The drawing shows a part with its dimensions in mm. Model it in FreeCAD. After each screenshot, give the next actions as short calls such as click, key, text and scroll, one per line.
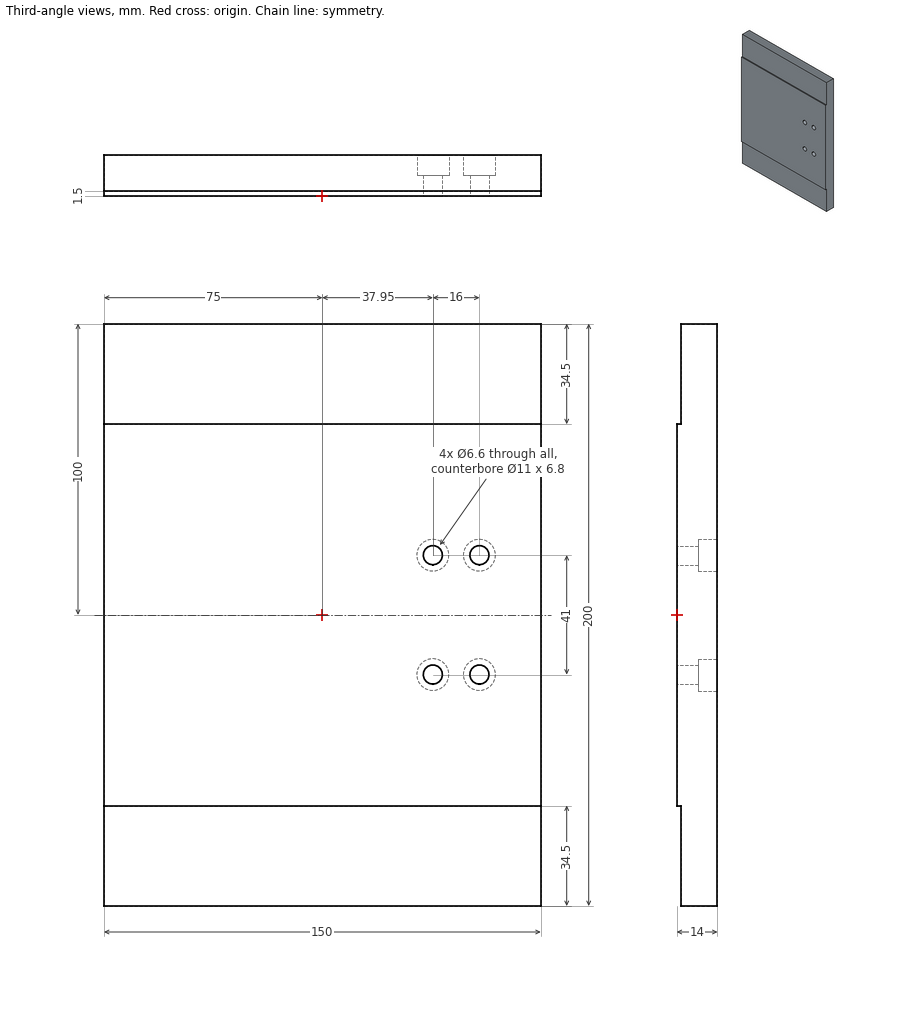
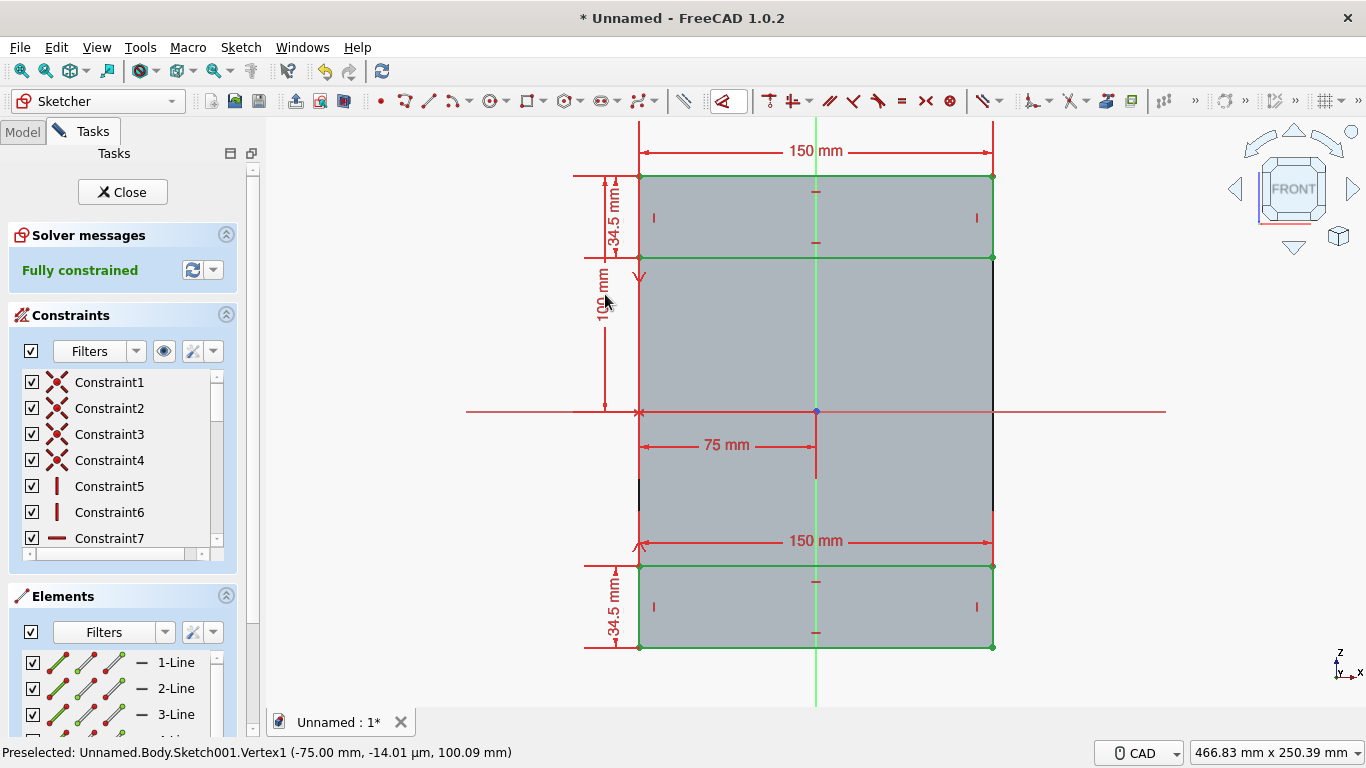
click(123, 192)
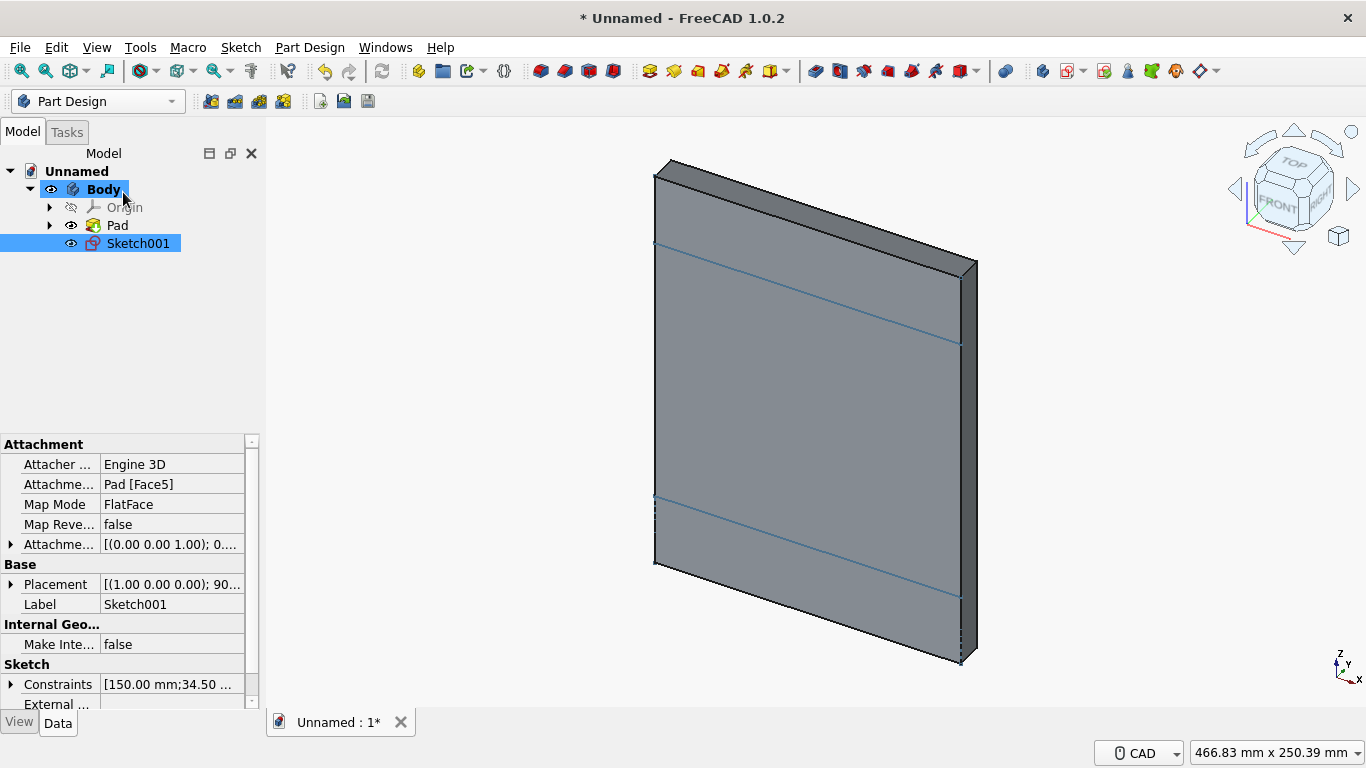
click(816, 72)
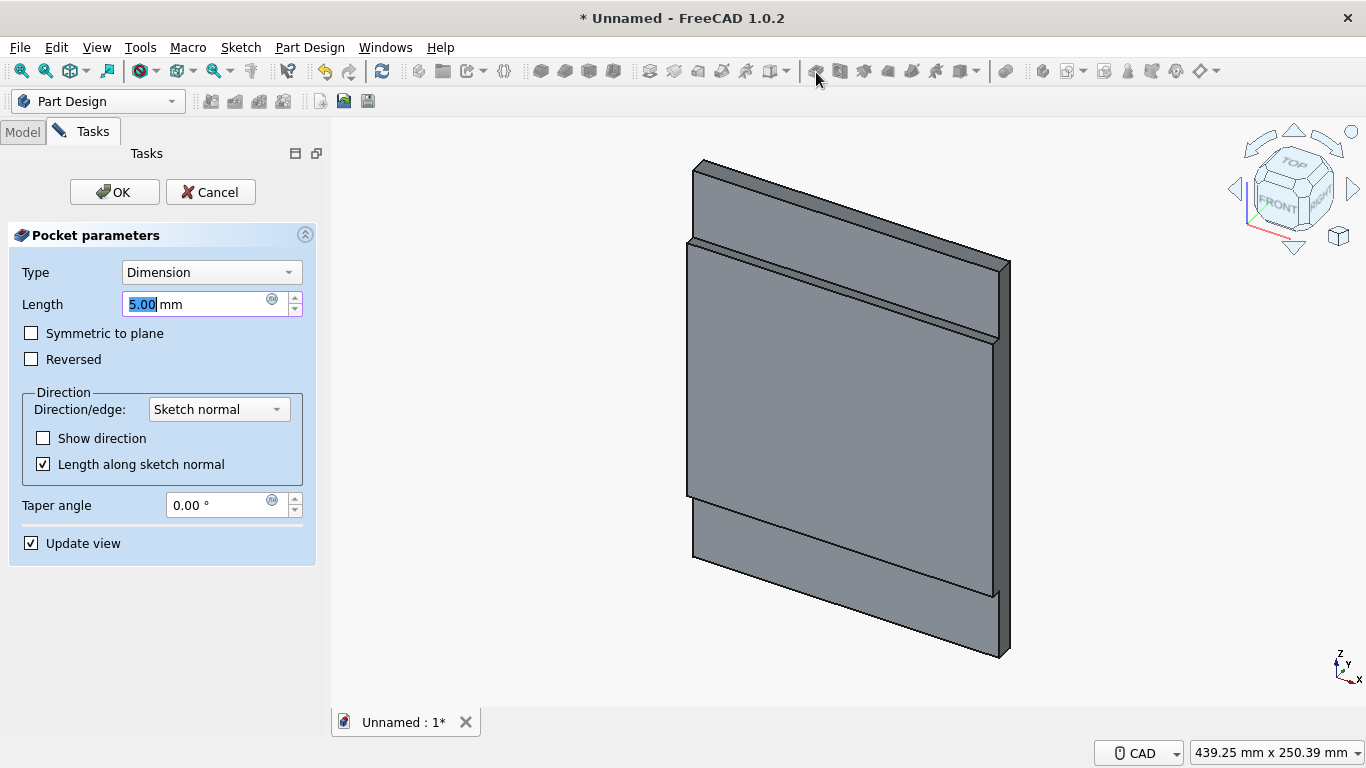
text(1.5)
key(Tab)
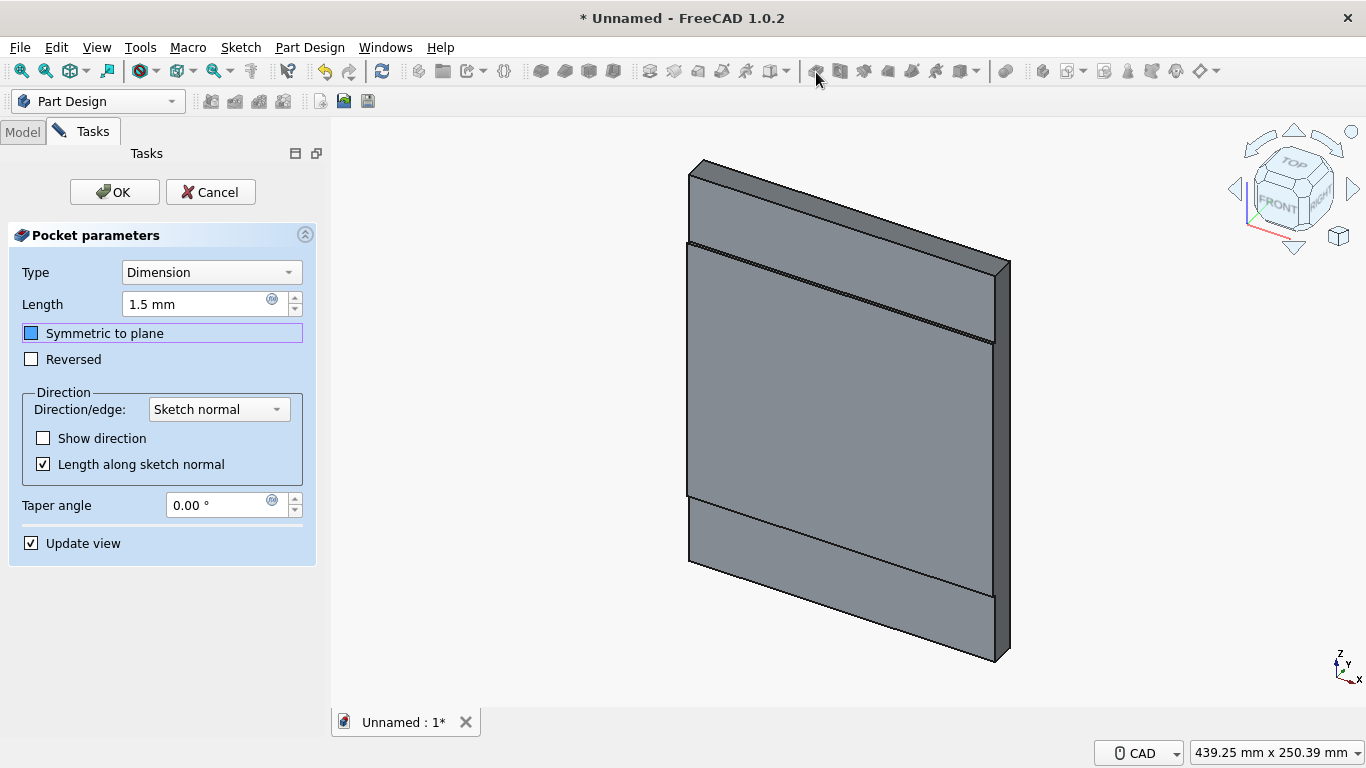
click(115, 192)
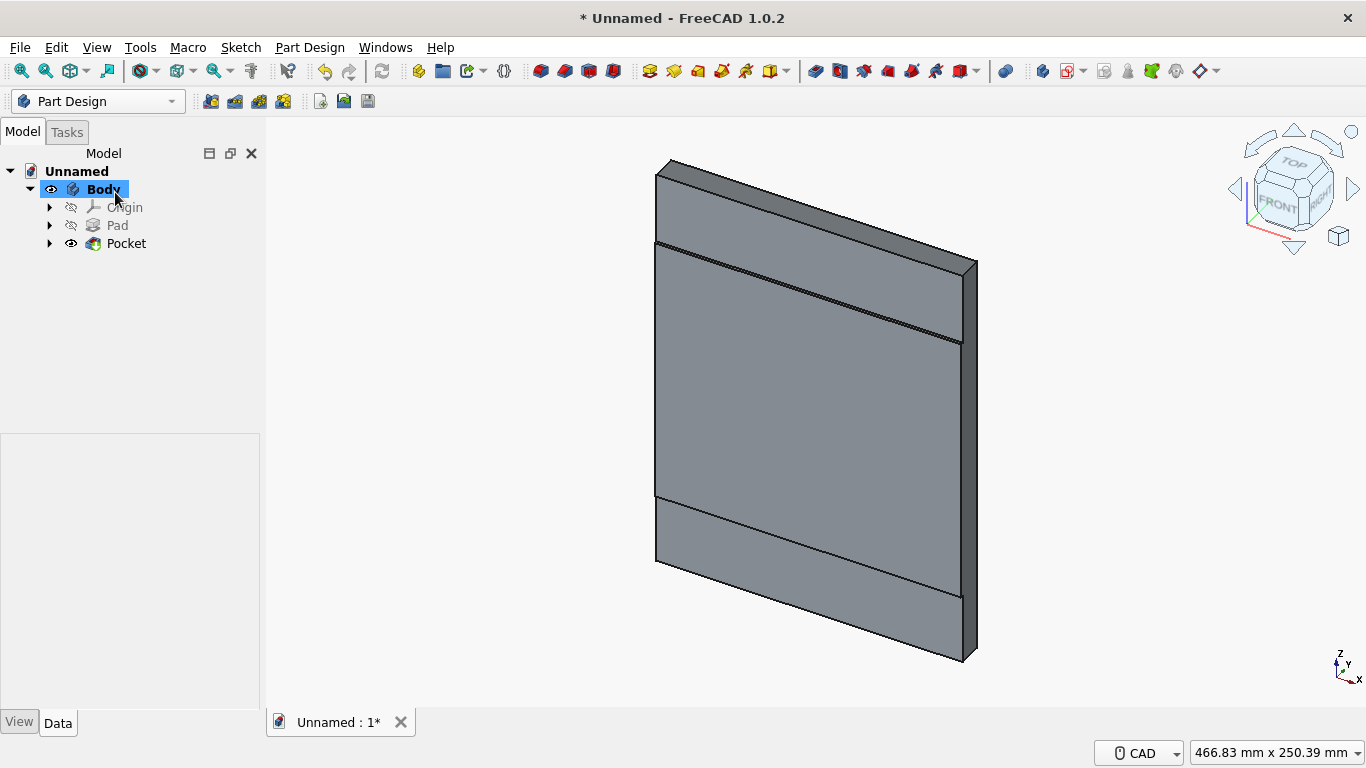
key(4)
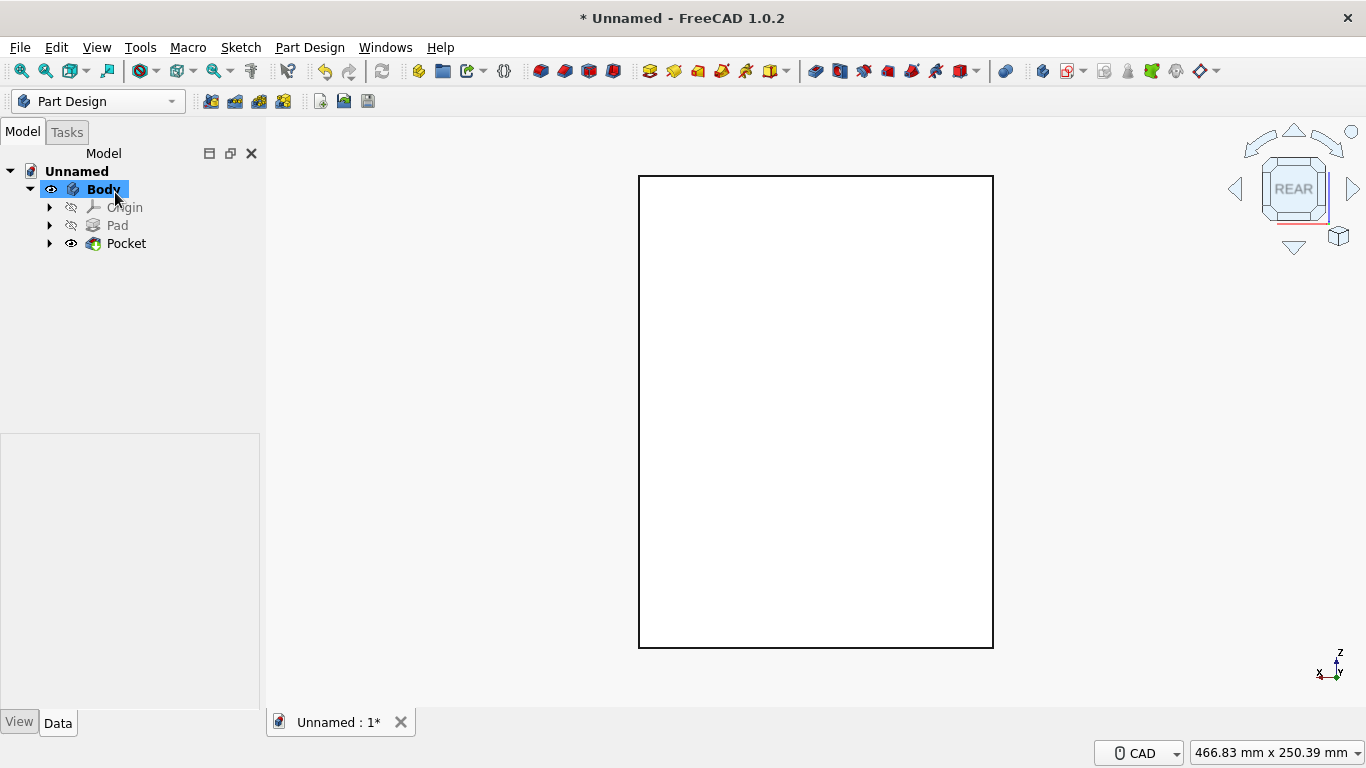
click(816, 411)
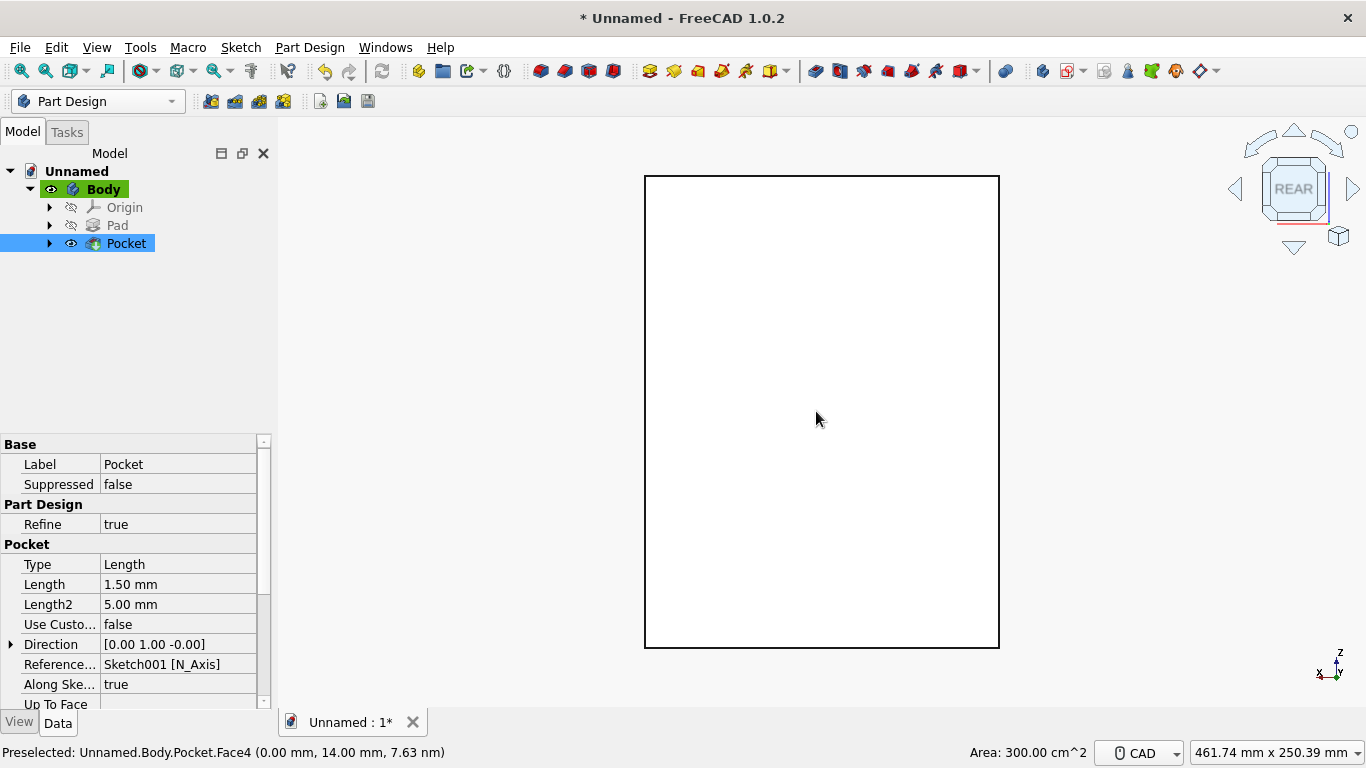
click(1068, 72)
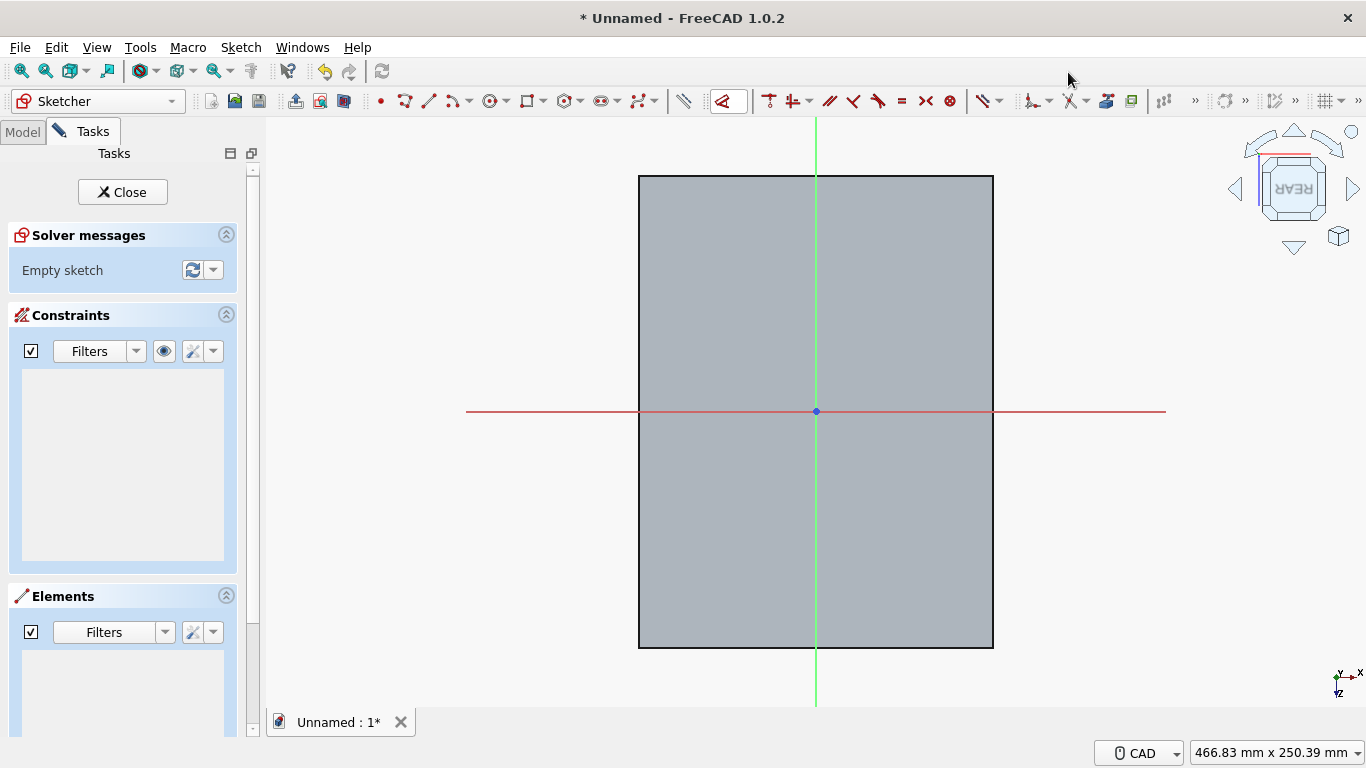
scroll(942, 412, up, 6)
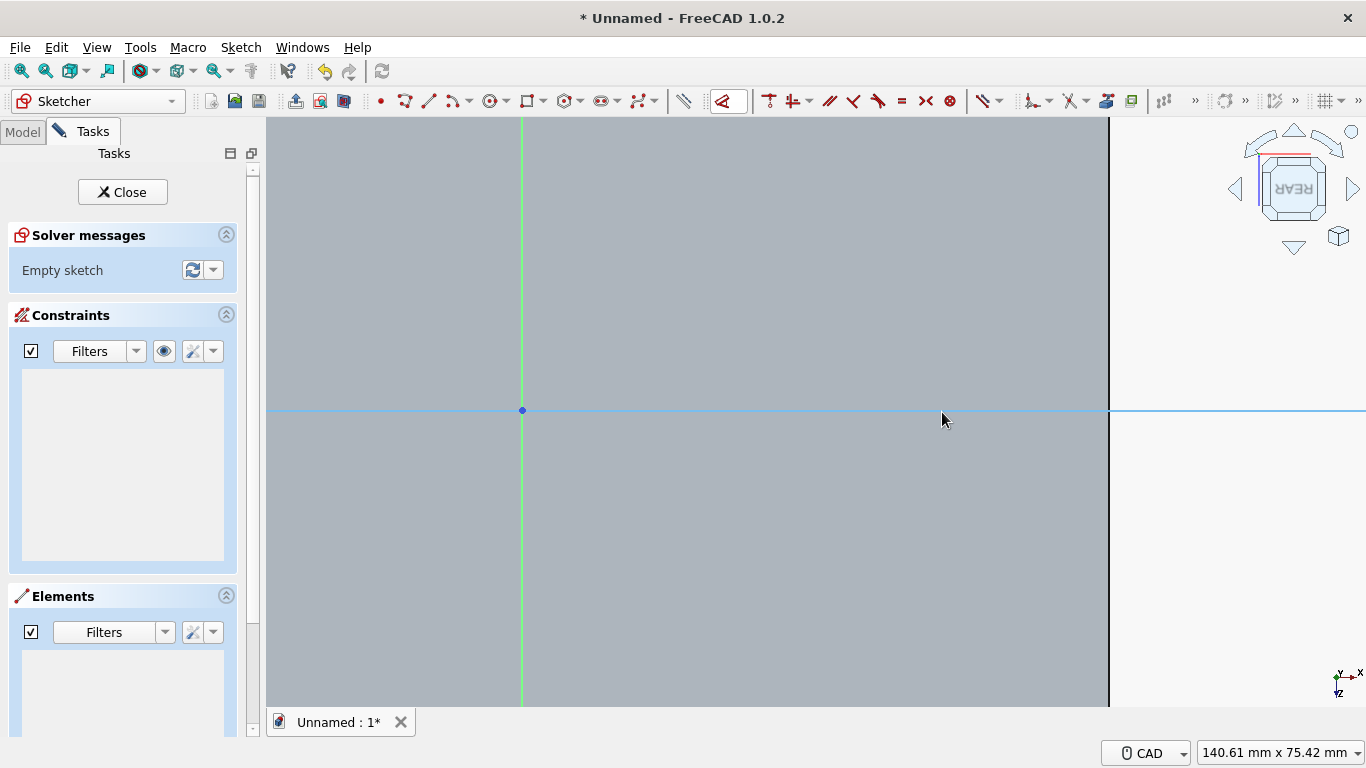
click(490, 102)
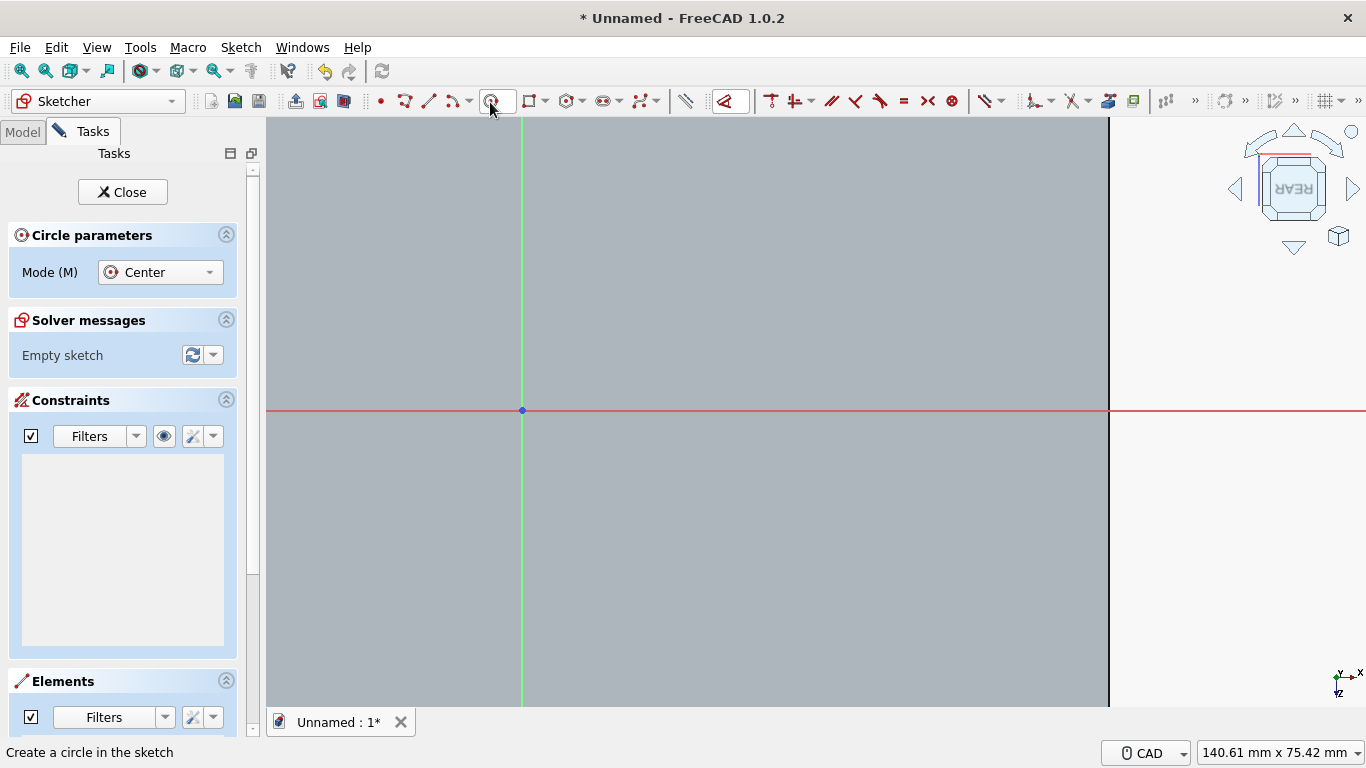
click(819, 571)
move(837, 553)